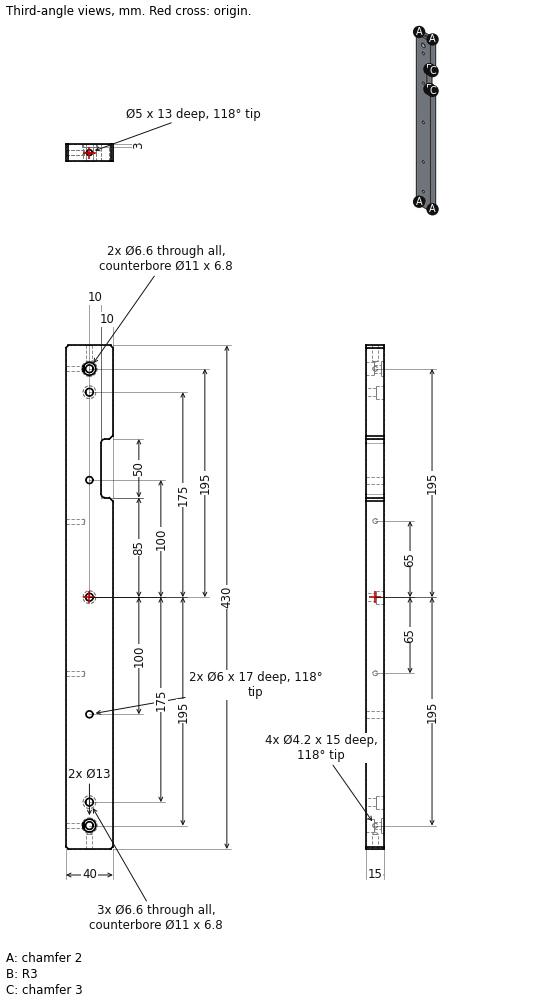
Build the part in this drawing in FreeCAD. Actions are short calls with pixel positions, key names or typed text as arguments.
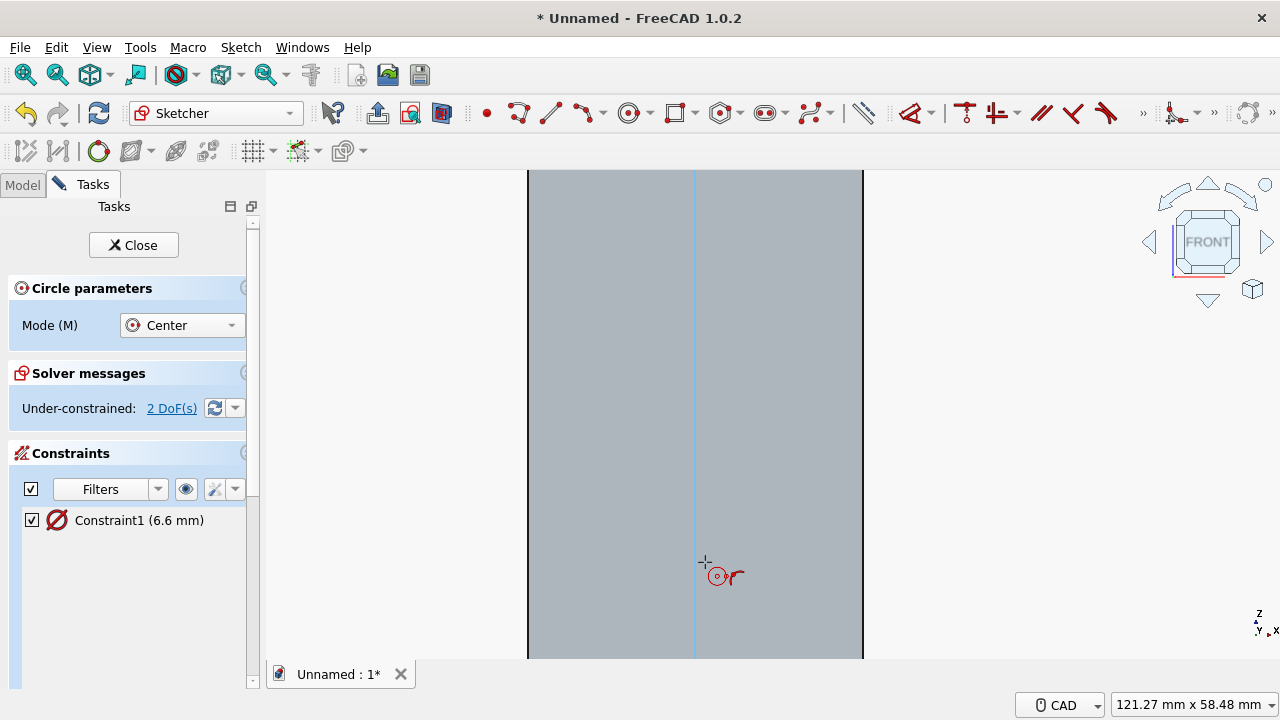
scroll(705, 563, down, 12)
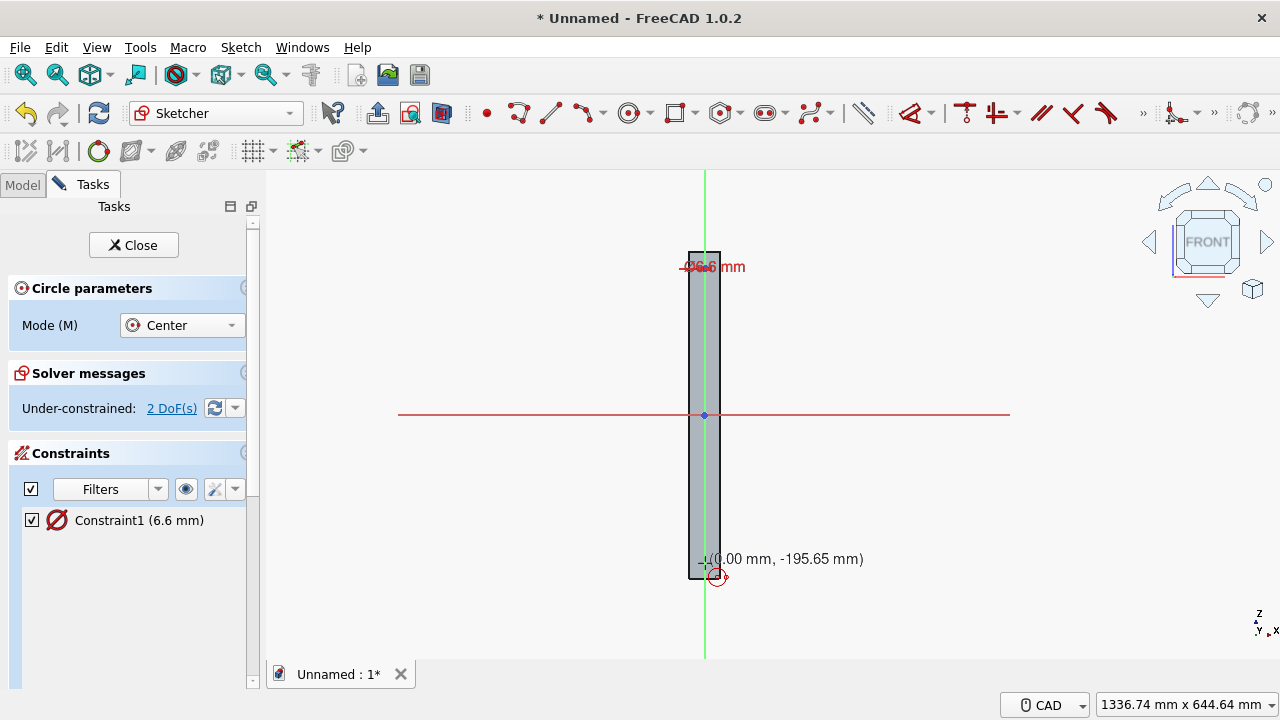
click(705, 563)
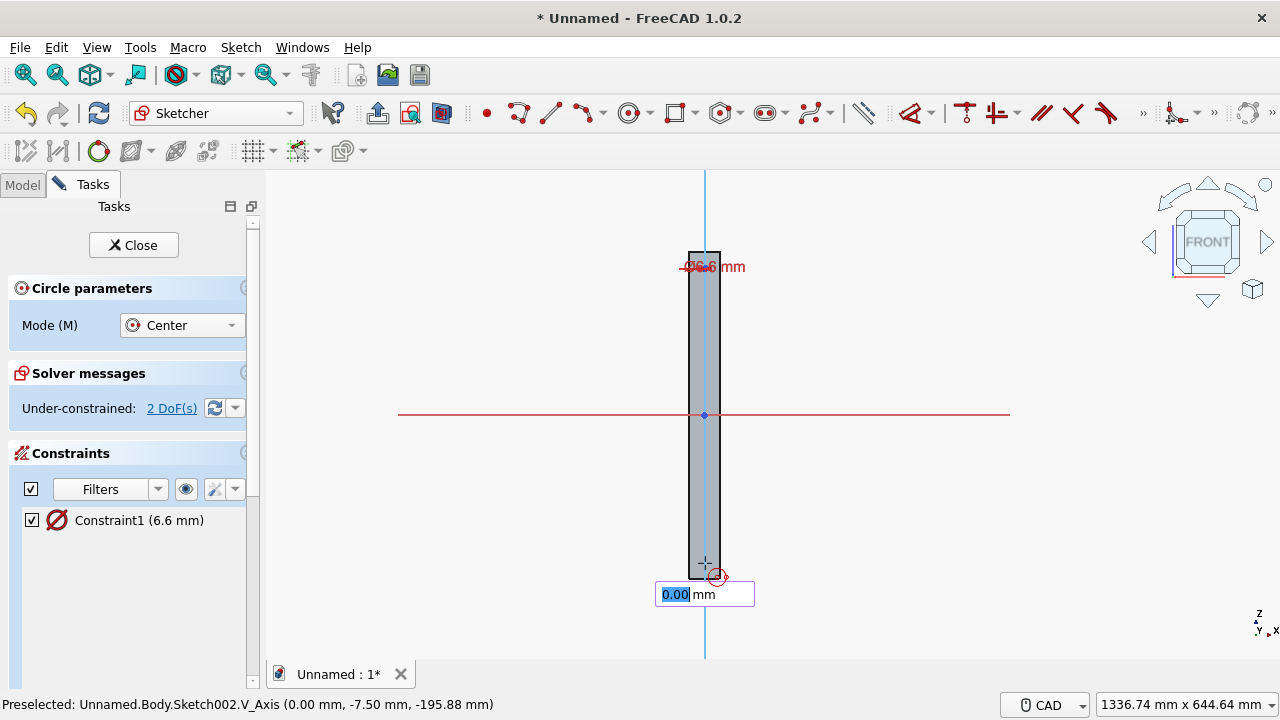
scroll(707, 562, up, 10)
move(703, 560)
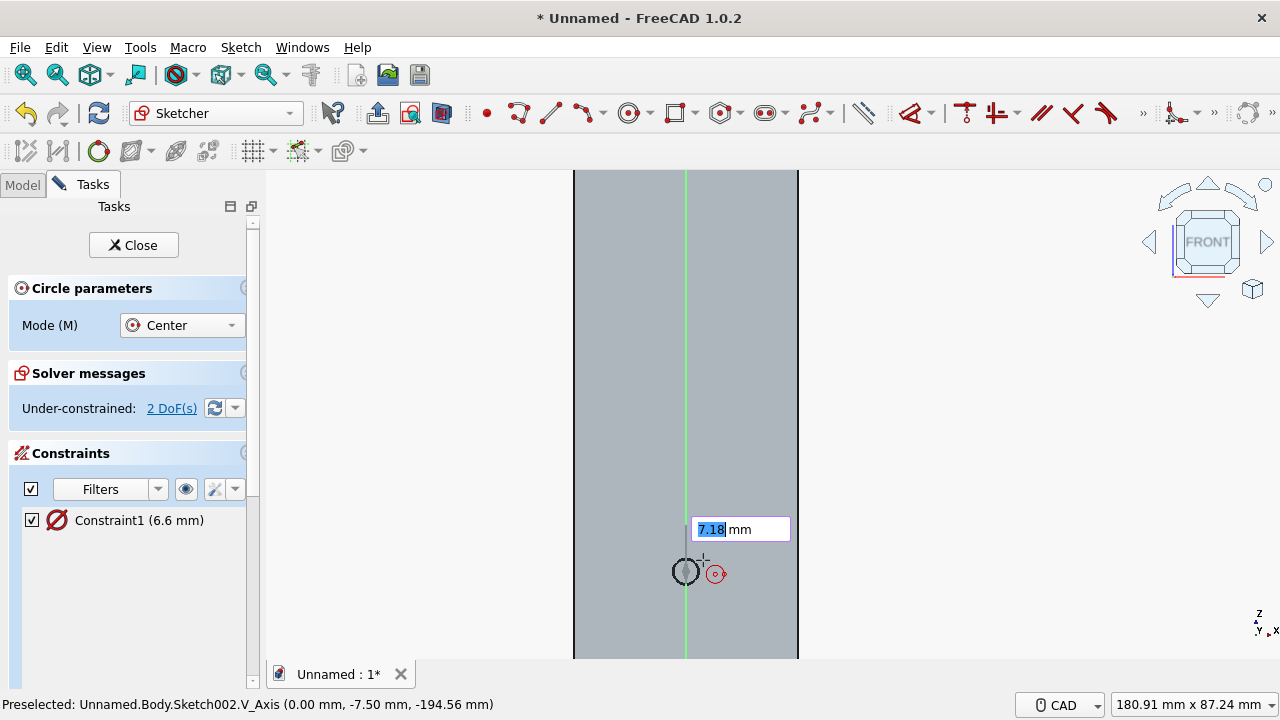
text(6.6)
key(Return)
key(Escape)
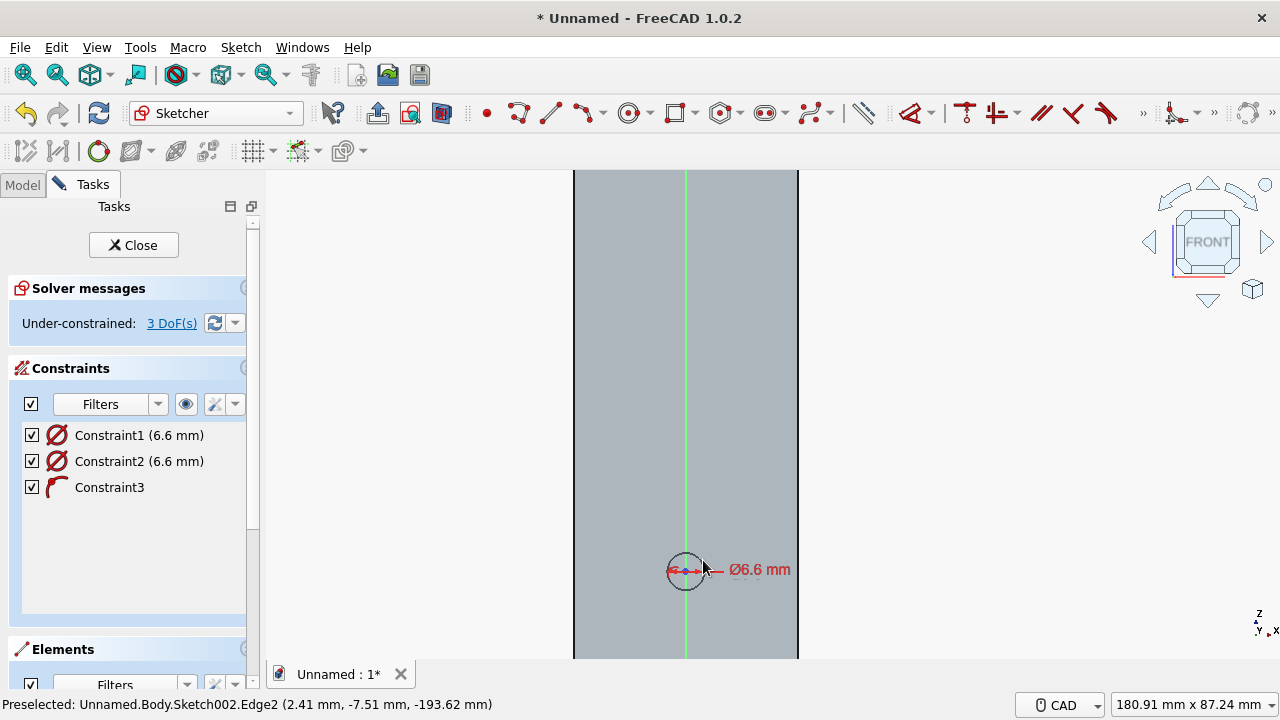
scroll(707, 562, down, 10)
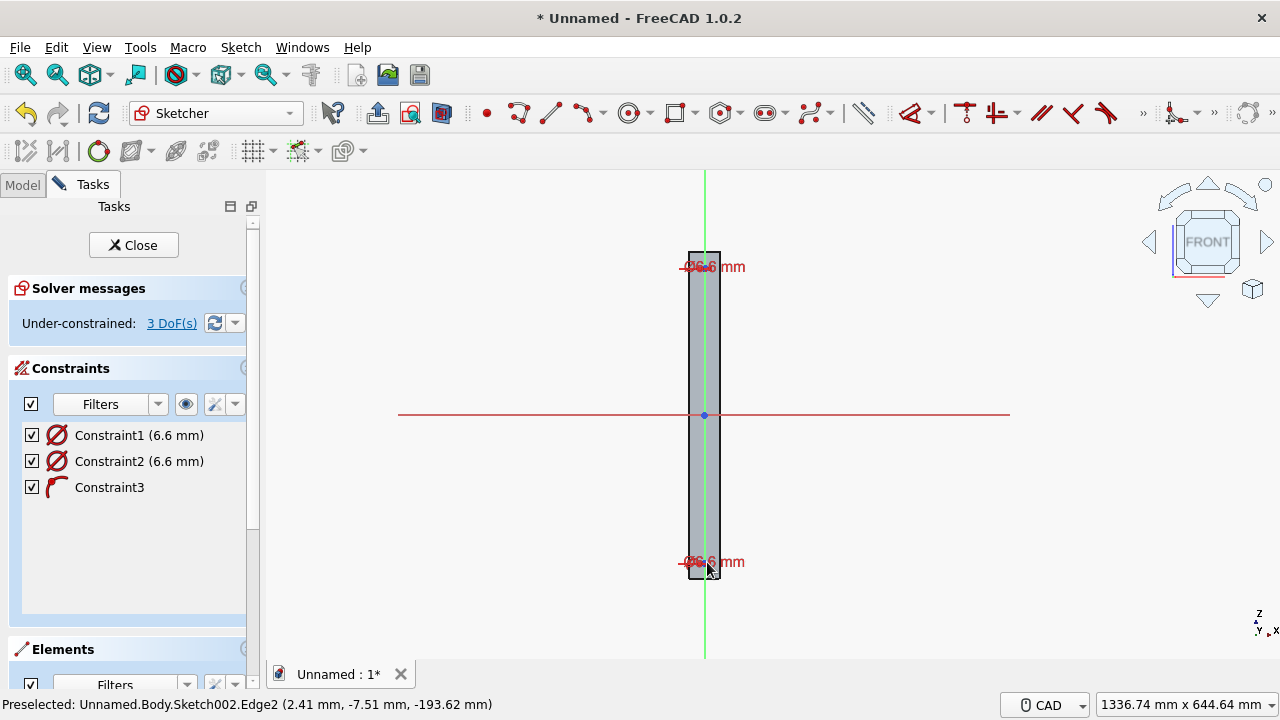
click(705, 269)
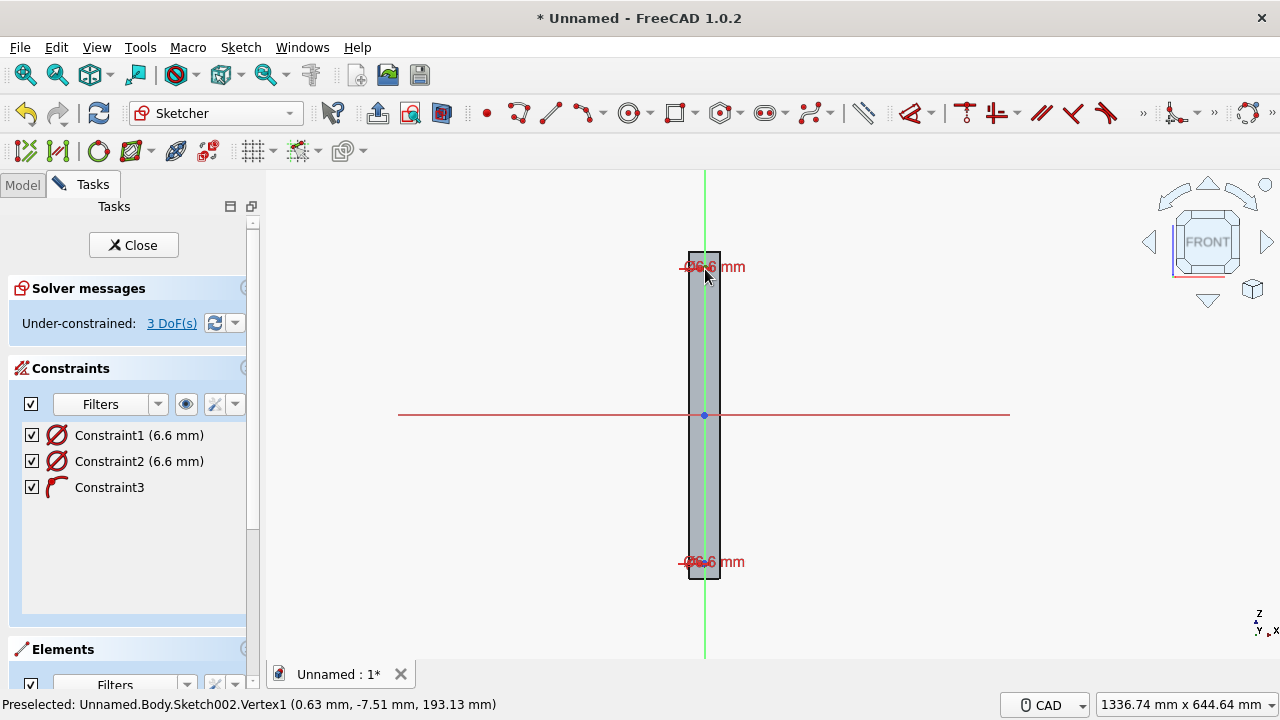
click(705, 600)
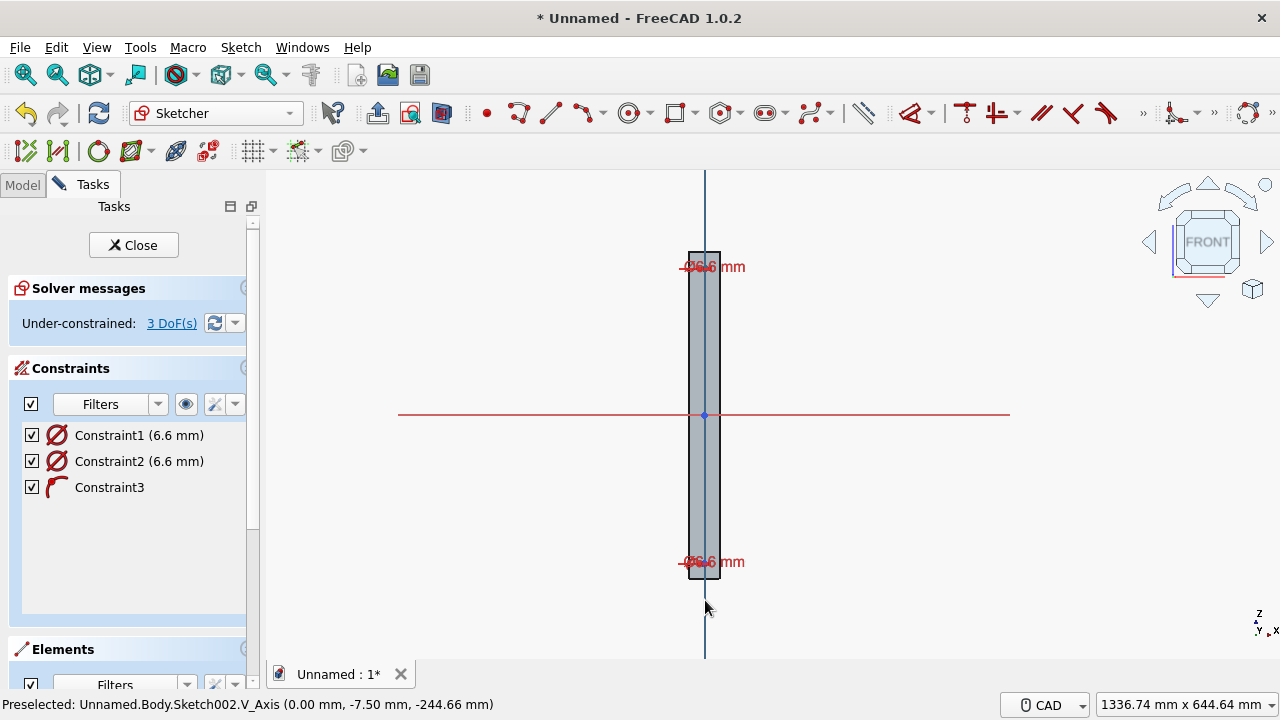
click(966, 114)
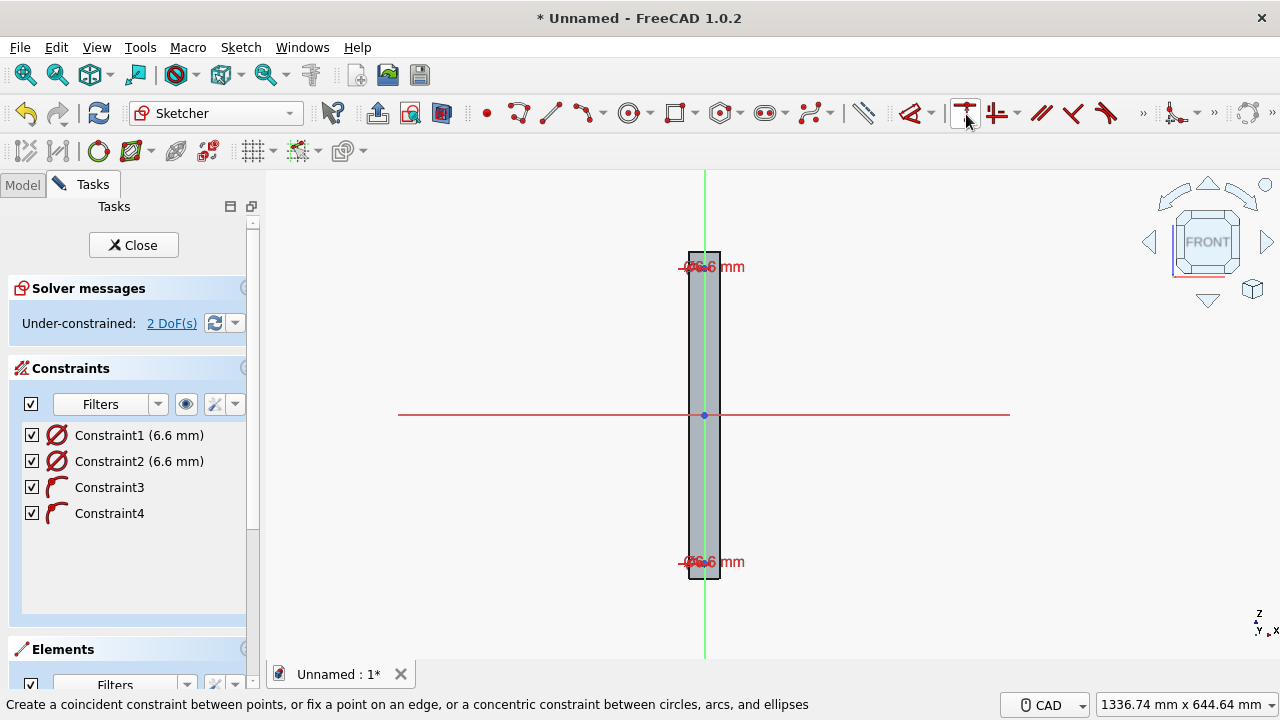
click(910, 114)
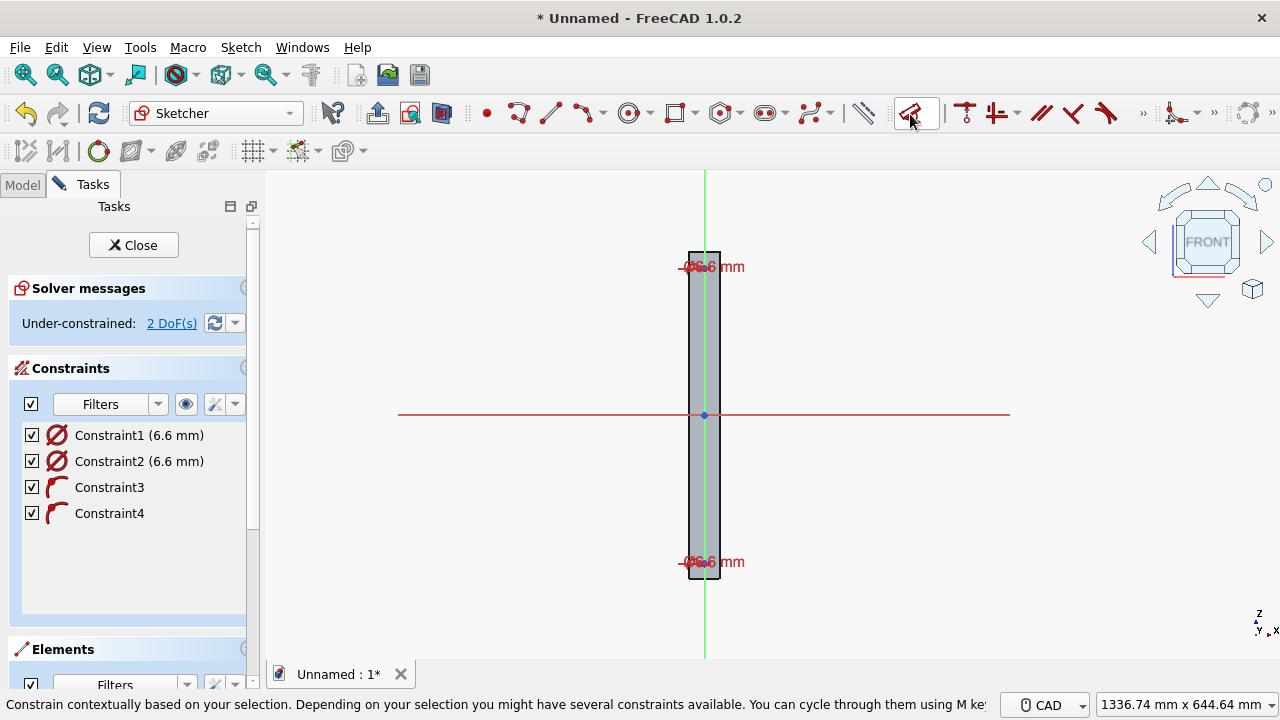
click(705, 269)
click(739, 342)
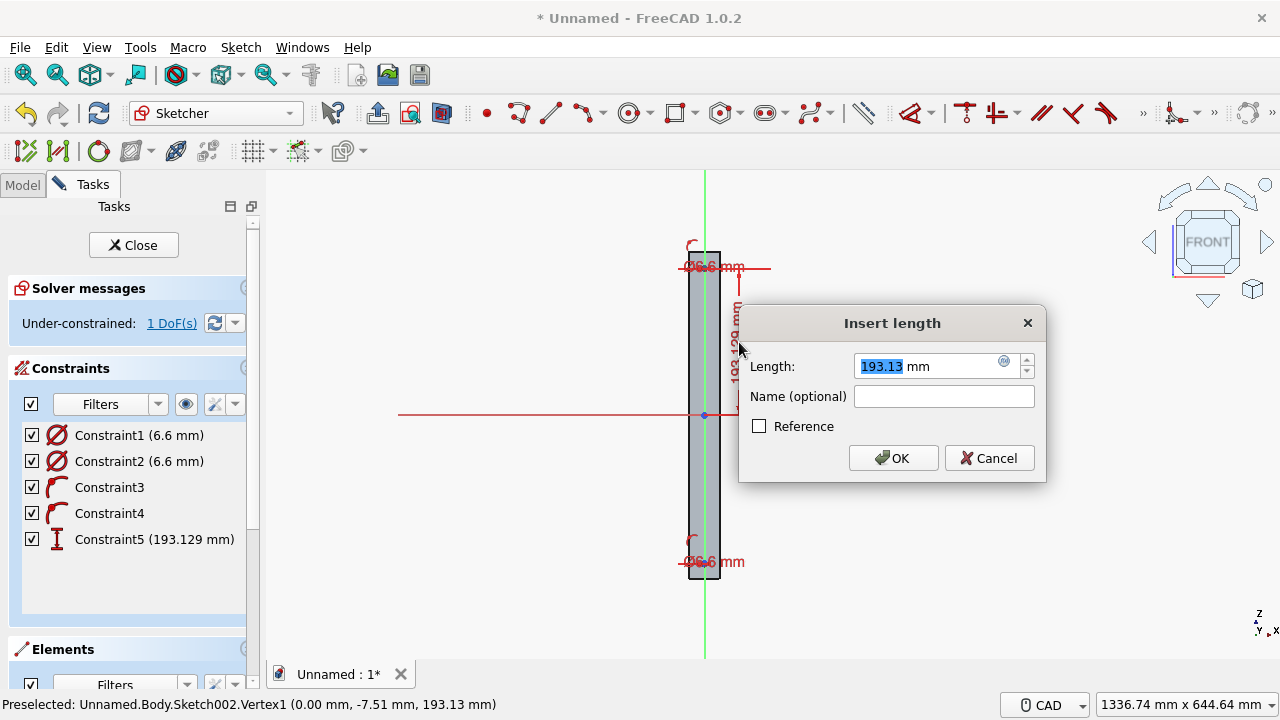
text(195)
key(Return)